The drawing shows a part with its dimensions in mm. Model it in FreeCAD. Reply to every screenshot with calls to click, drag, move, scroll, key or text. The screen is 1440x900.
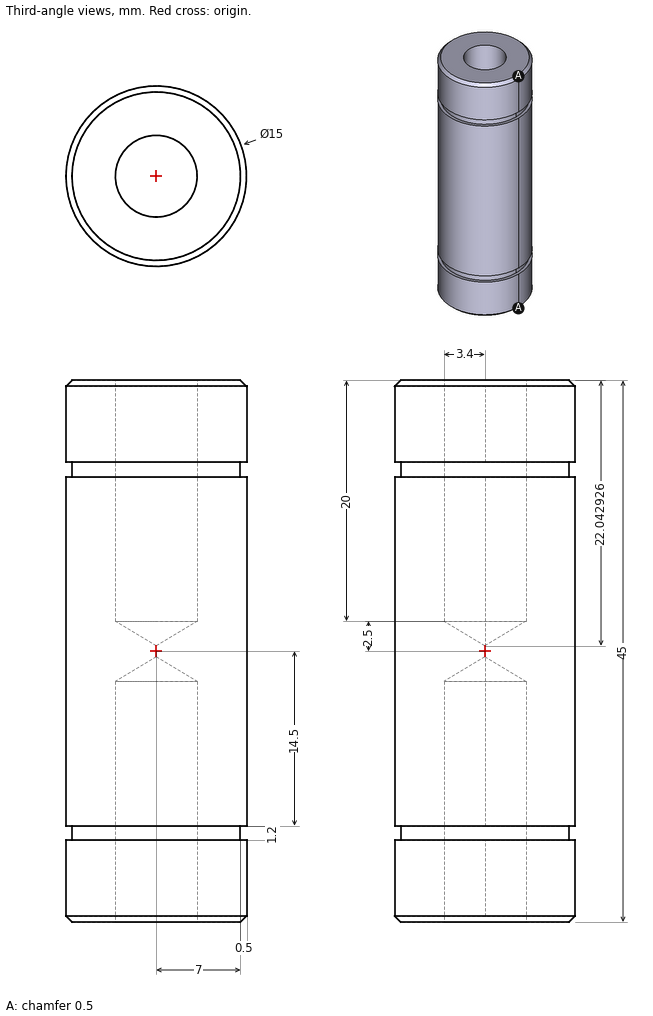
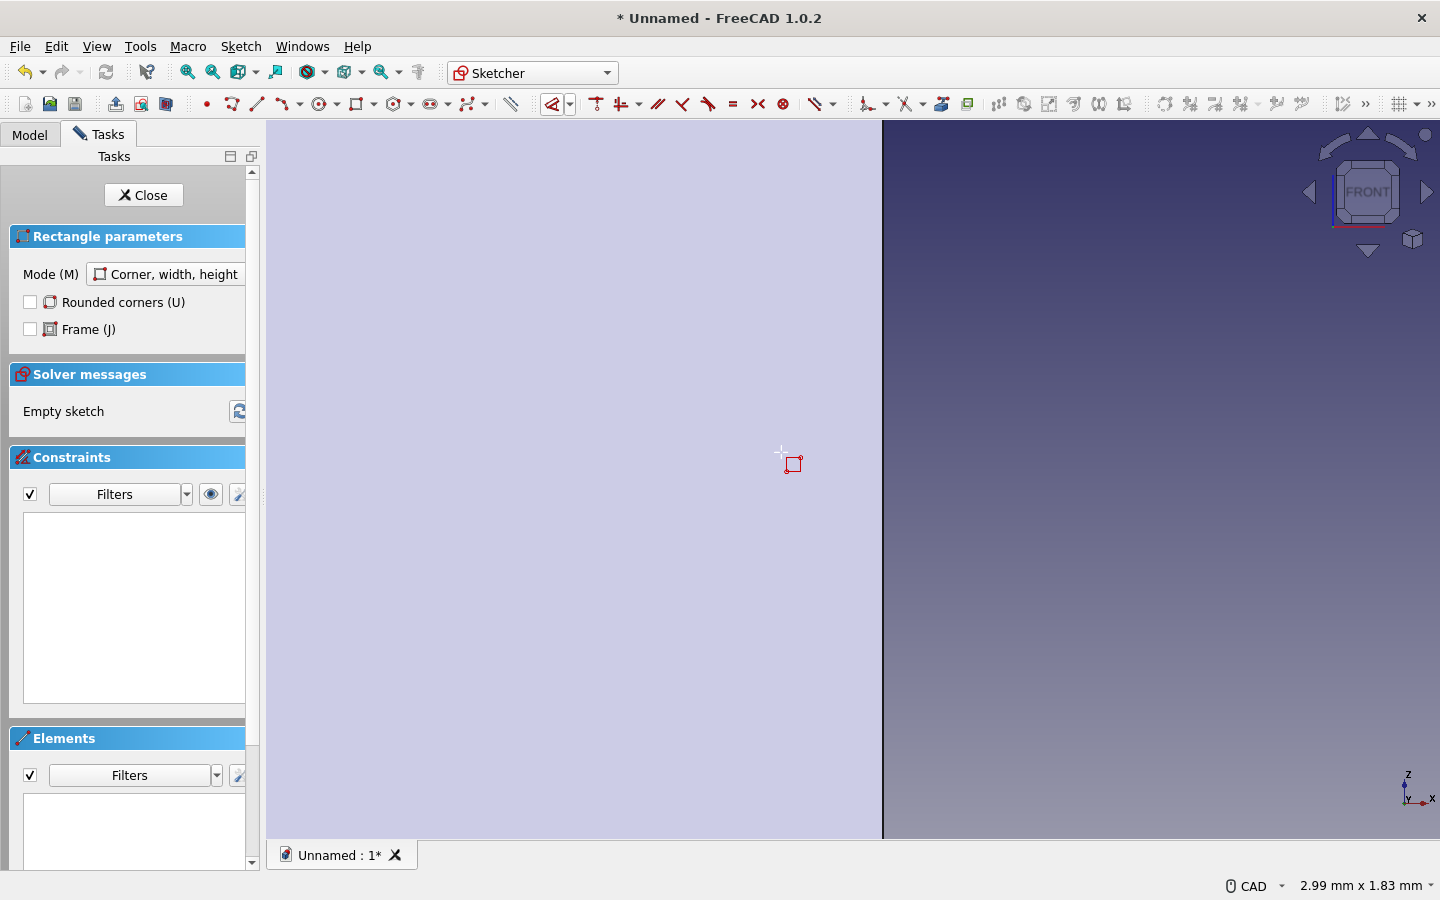
click(686, 244)
click(883, 715)
key(Escape)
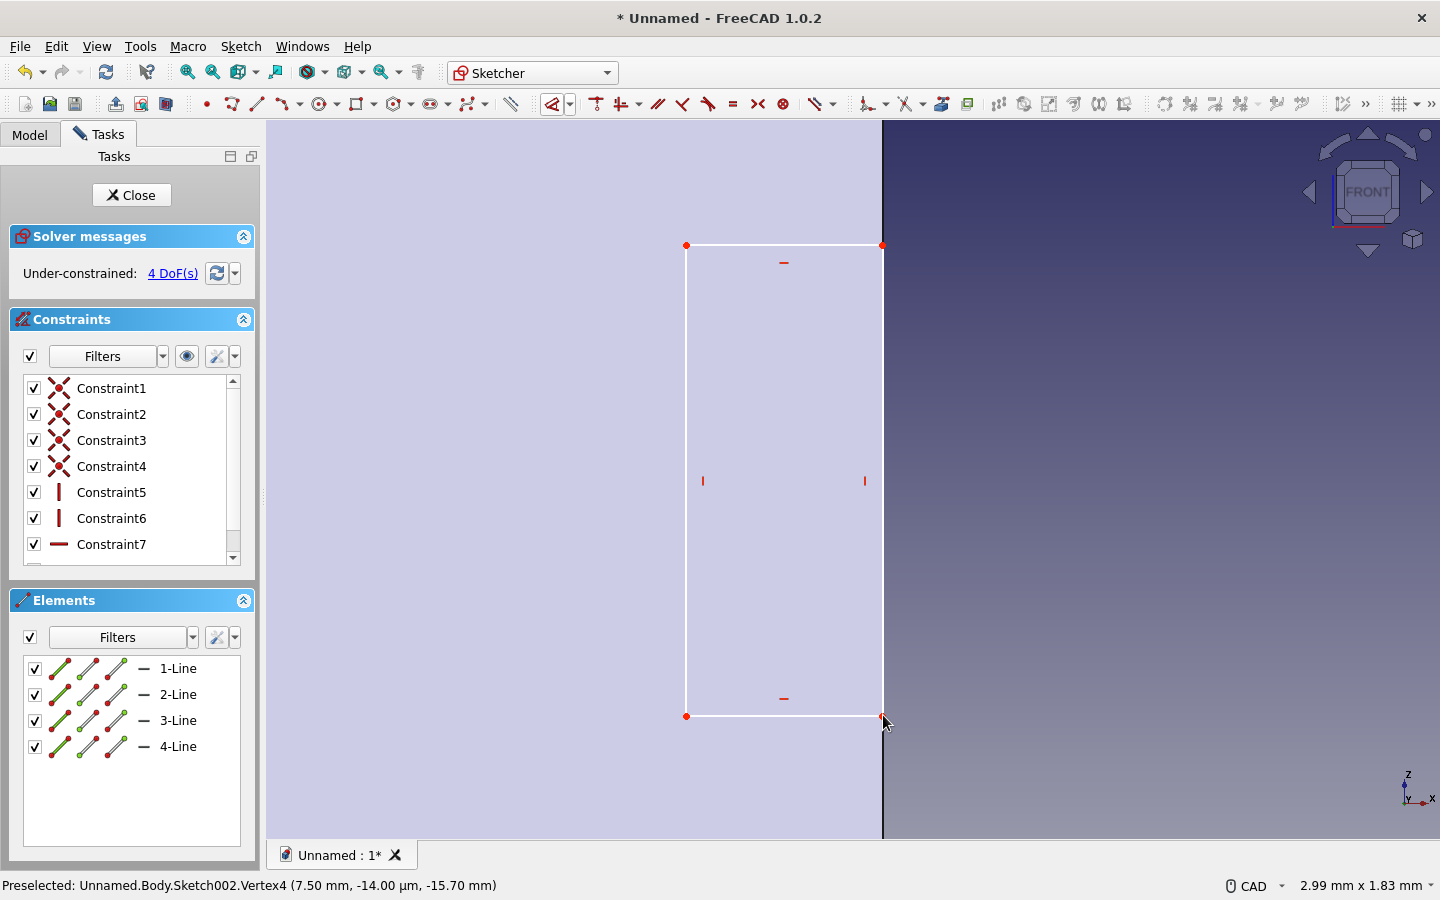
click(686, 245)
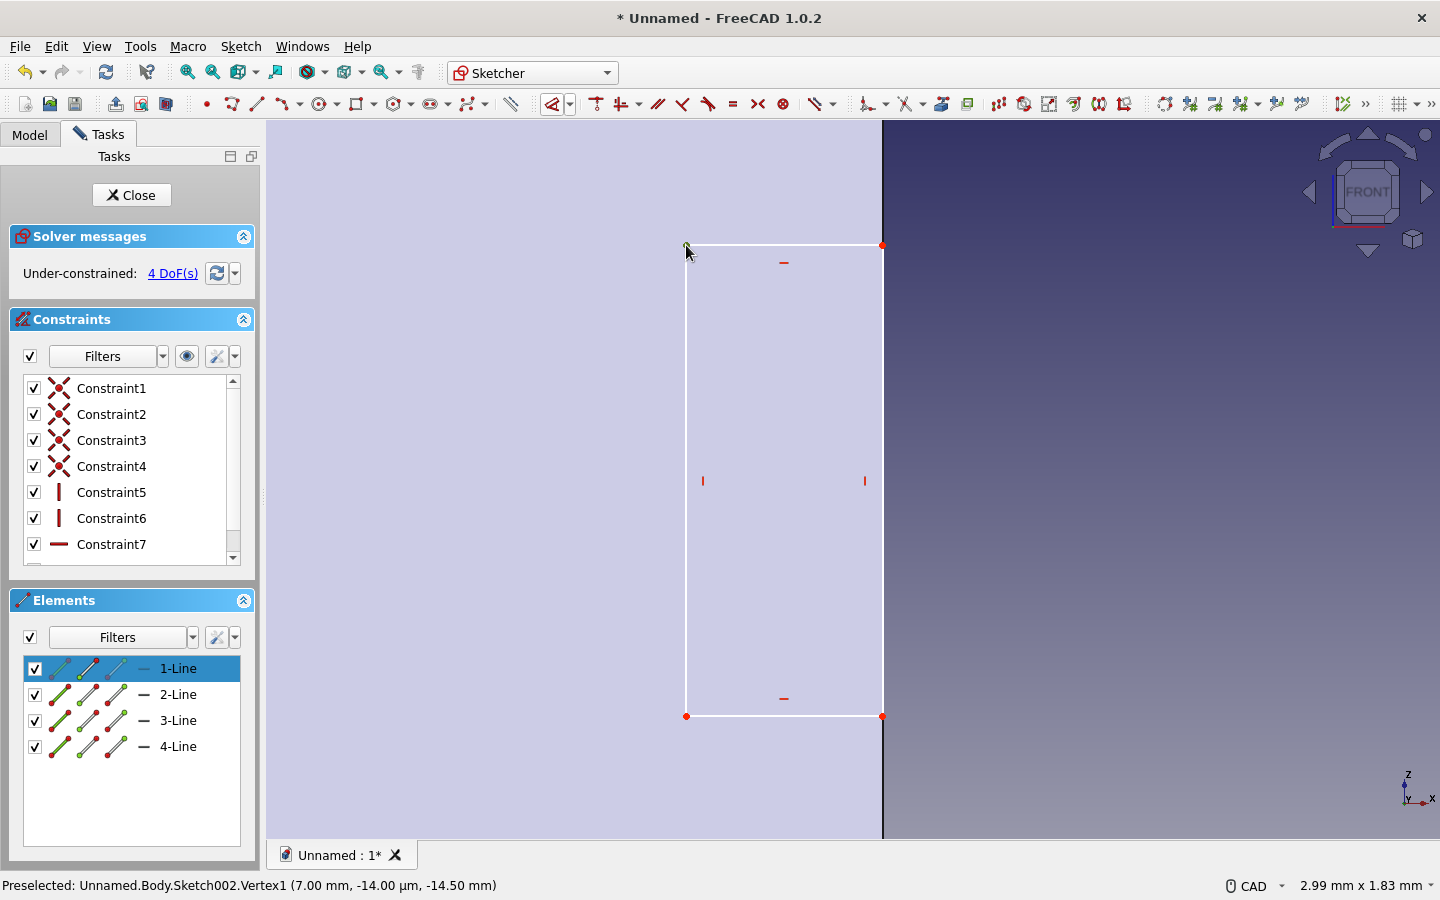
key(l)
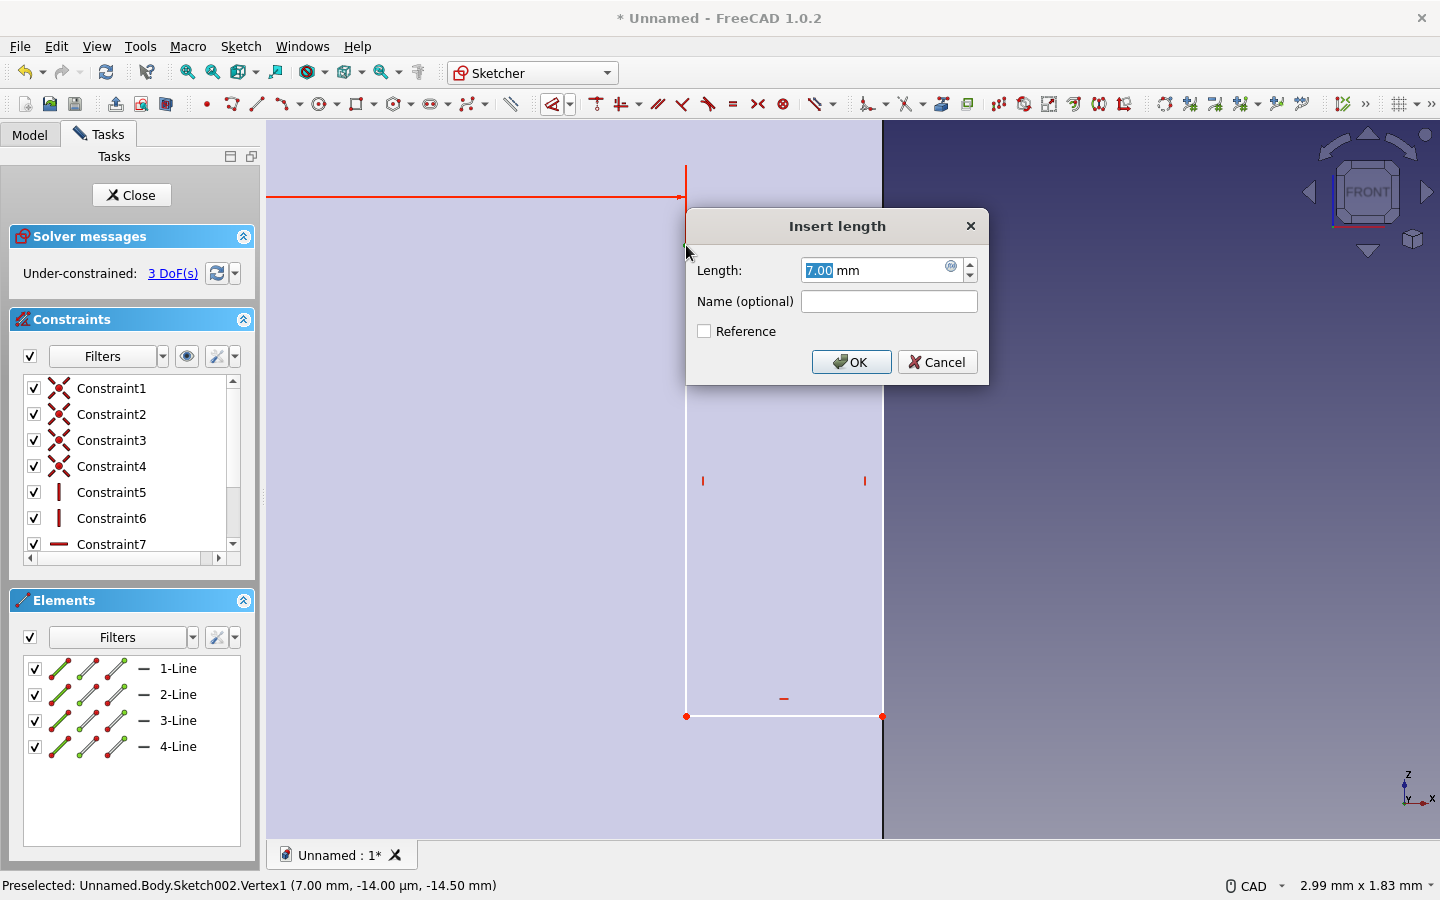
text(7)
key(Return)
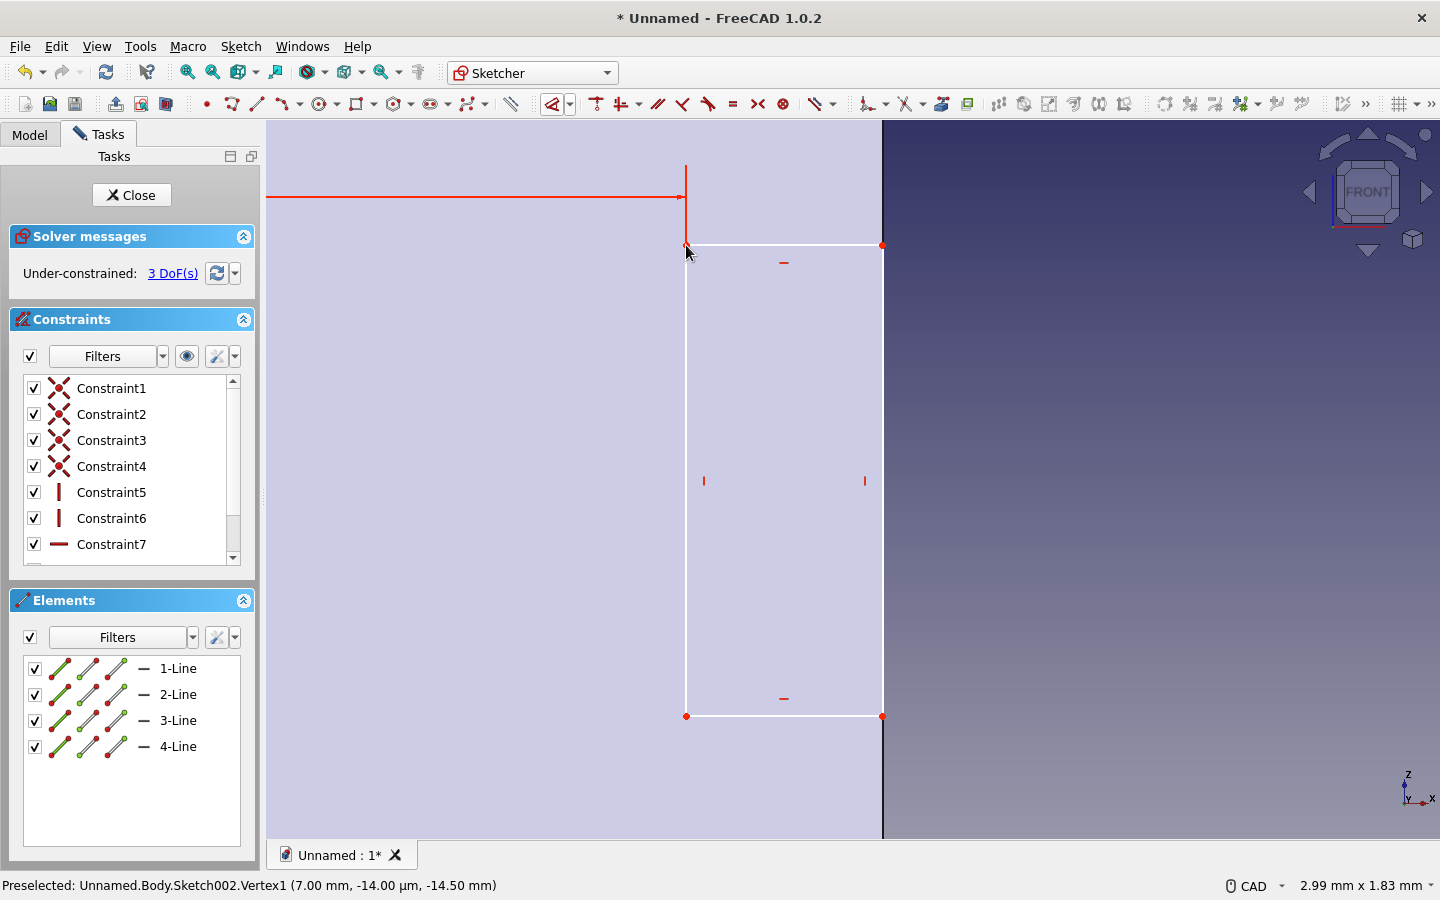
click(686, 386)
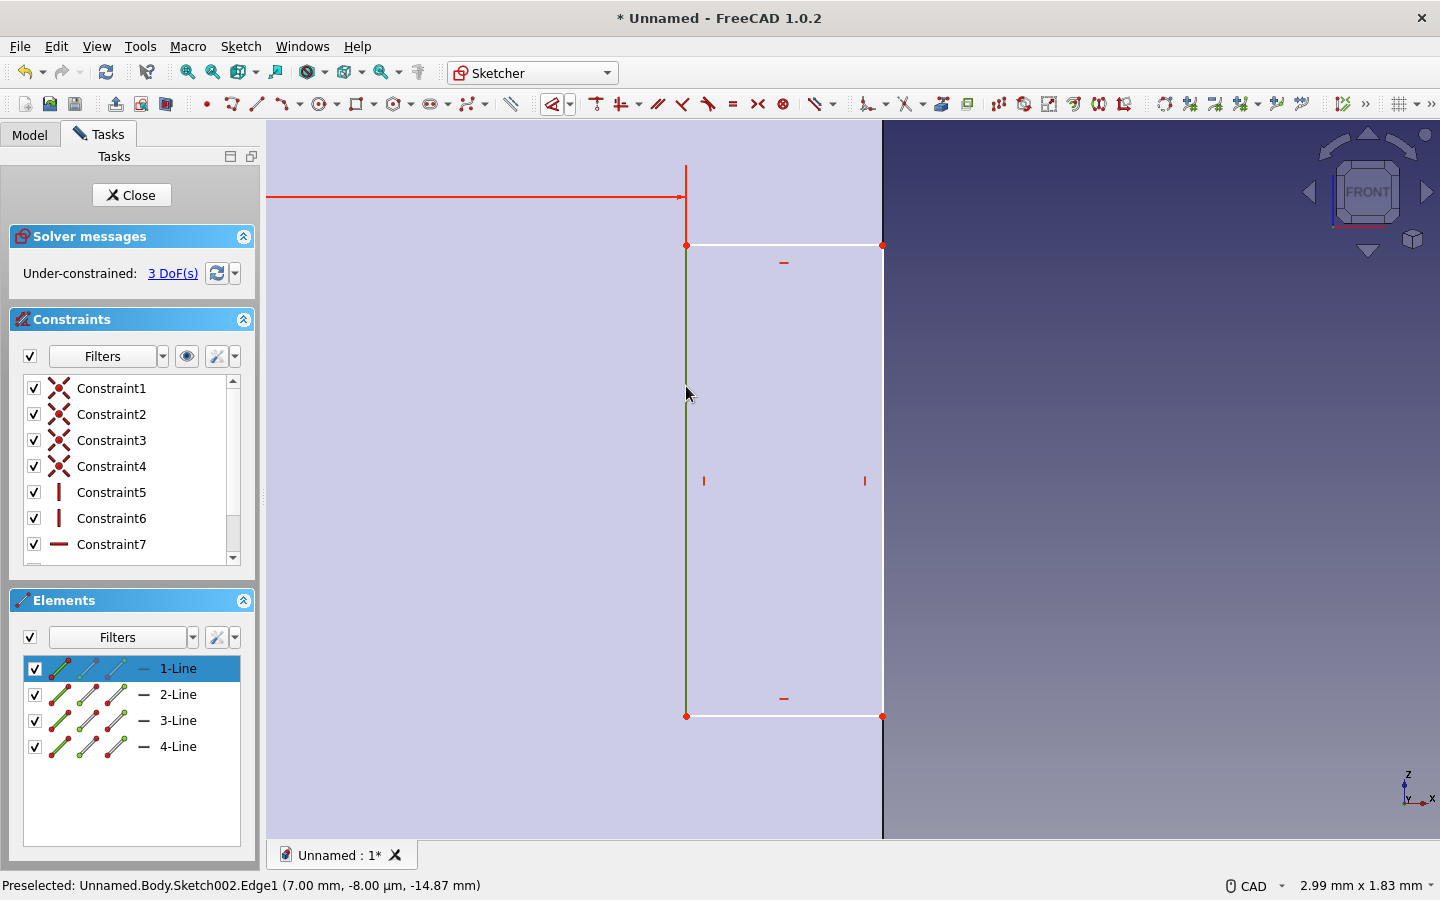
key(i)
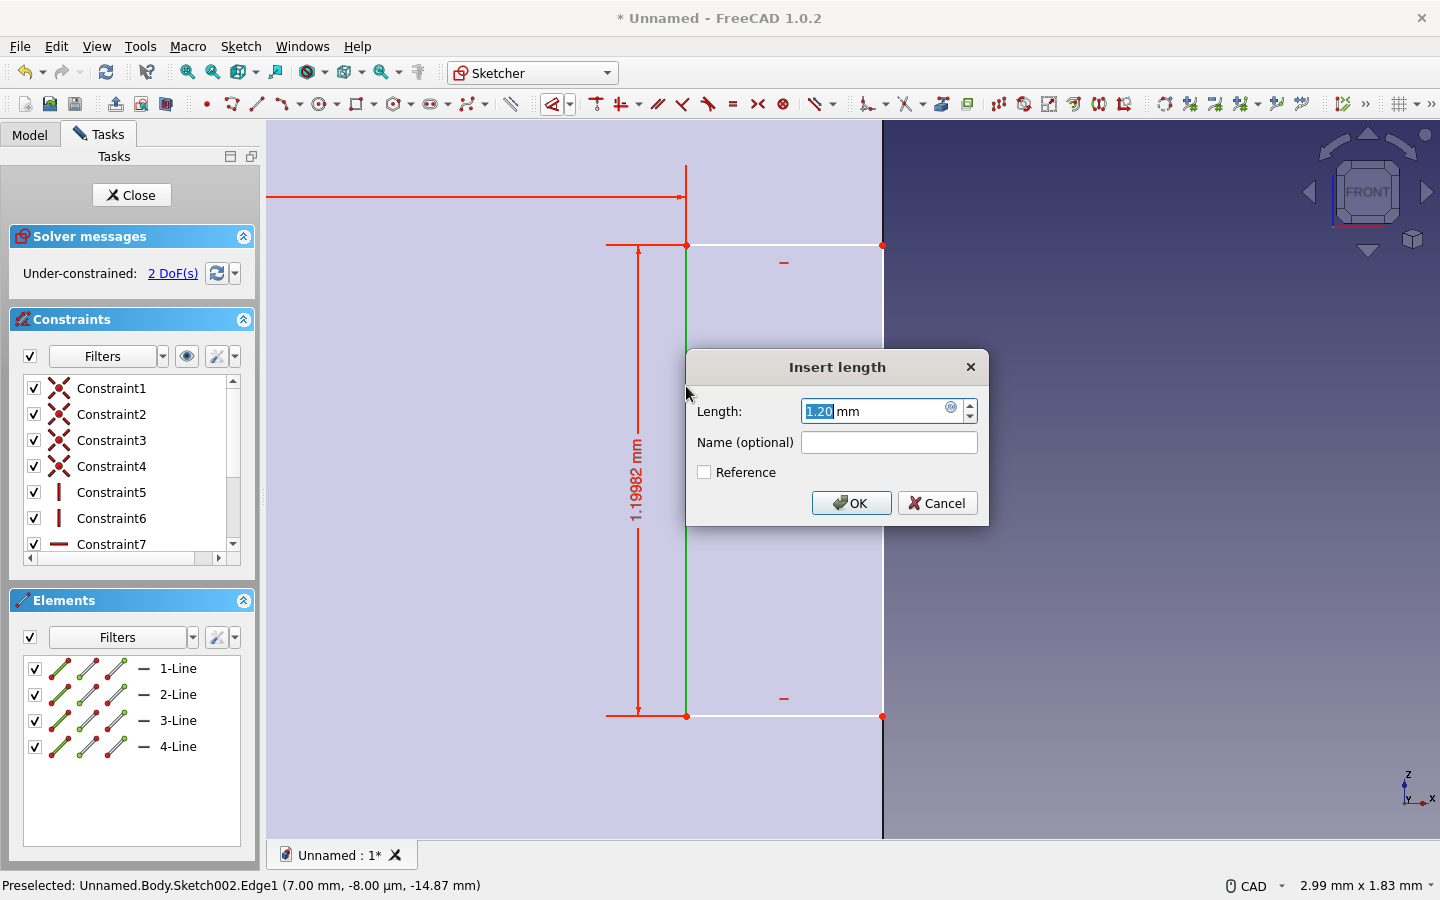
text(1.2)
key(Return)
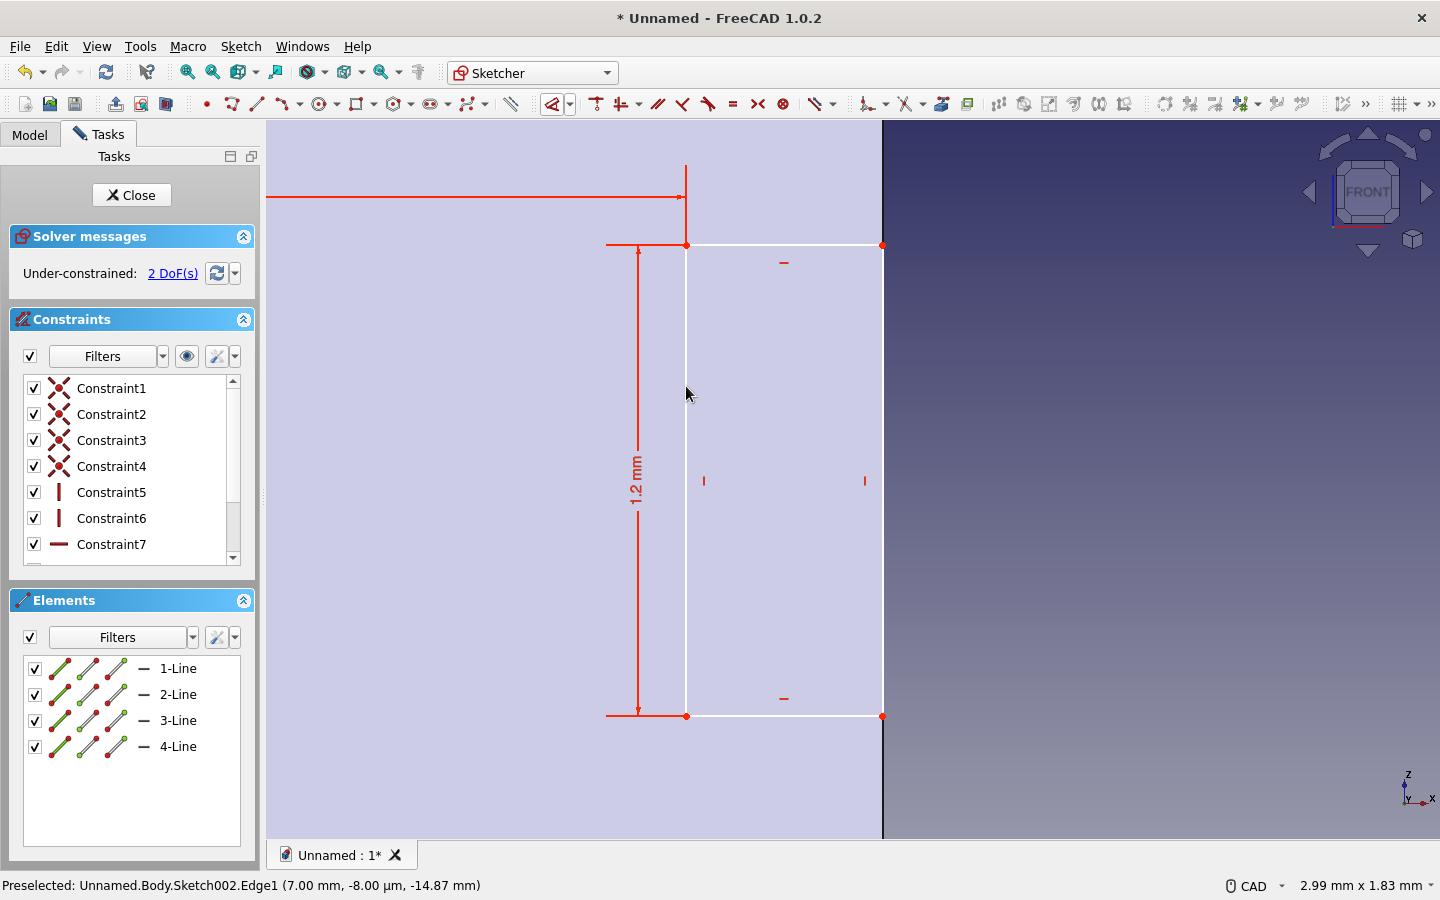
click(745, 716)